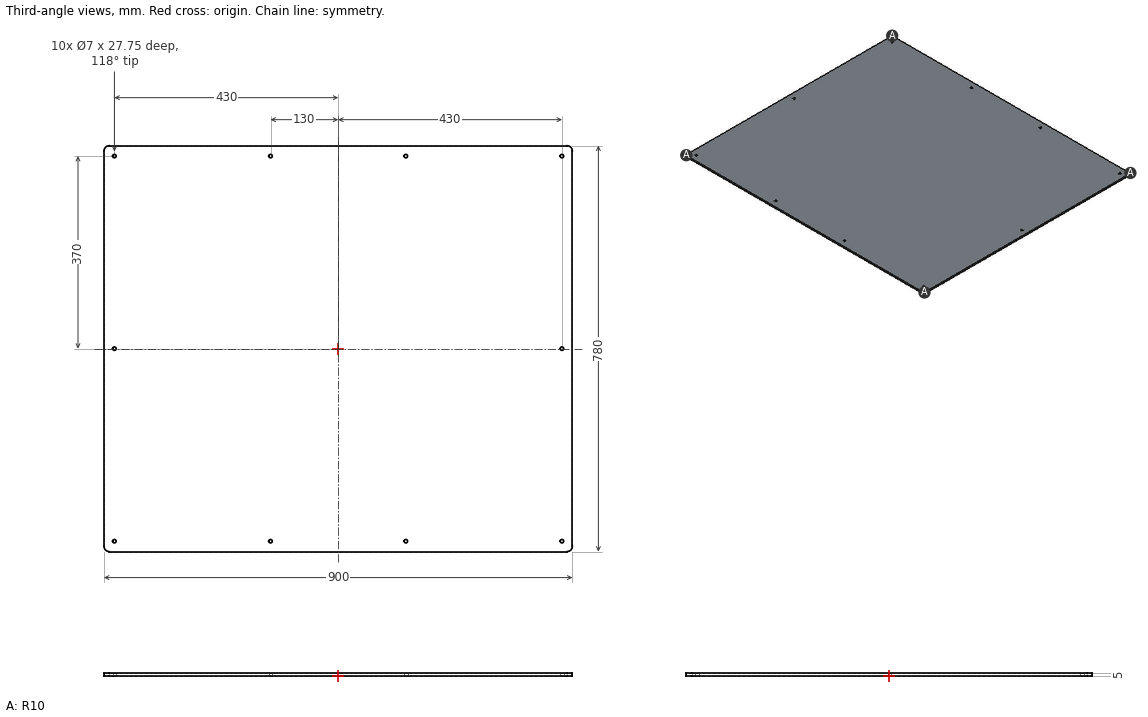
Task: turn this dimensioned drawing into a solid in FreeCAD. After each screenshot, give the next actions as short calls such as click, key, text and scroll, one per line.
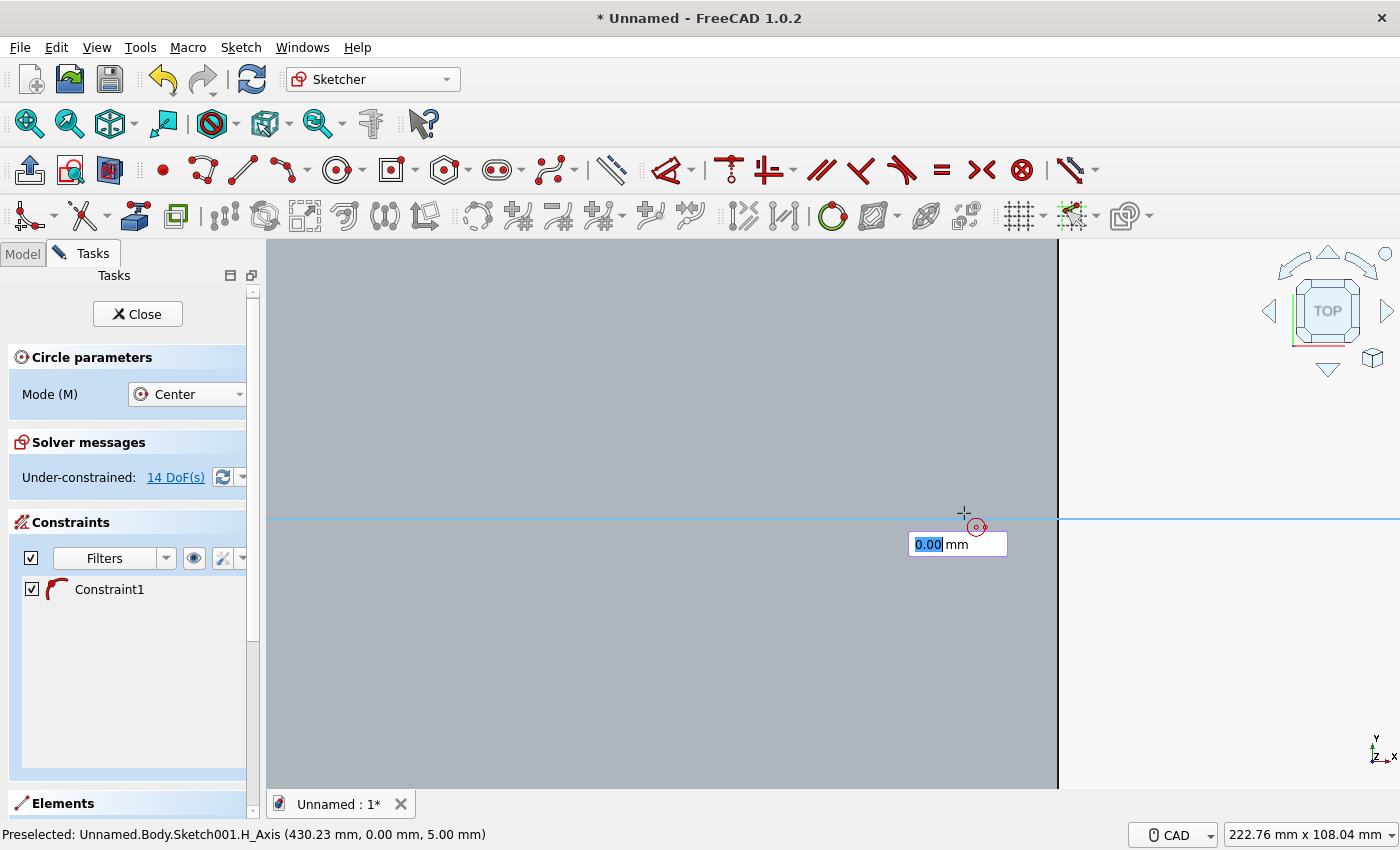
click(963, 503)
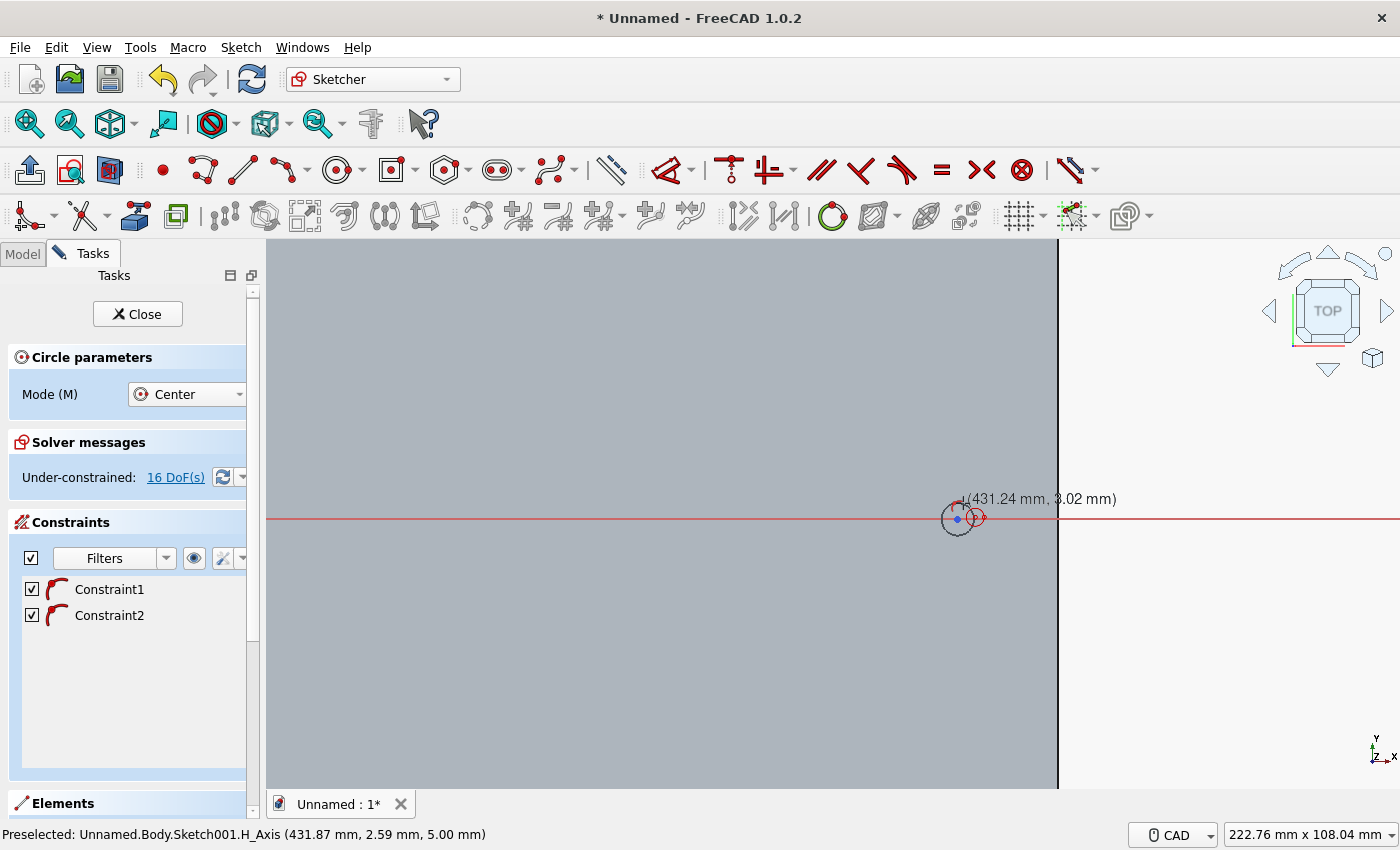
scroll(964, 513, down, 12)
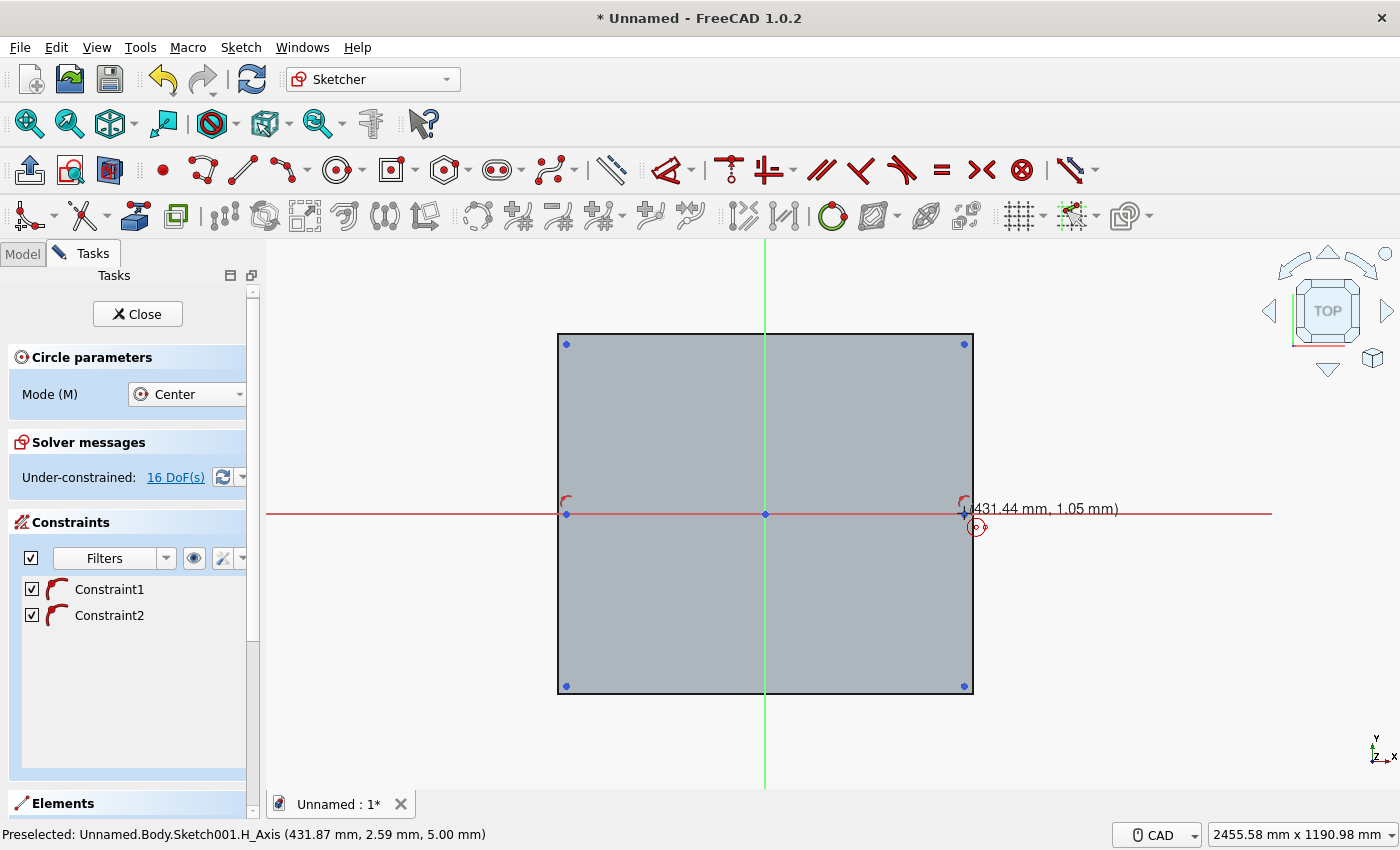
scroll(705, 343, up, 14)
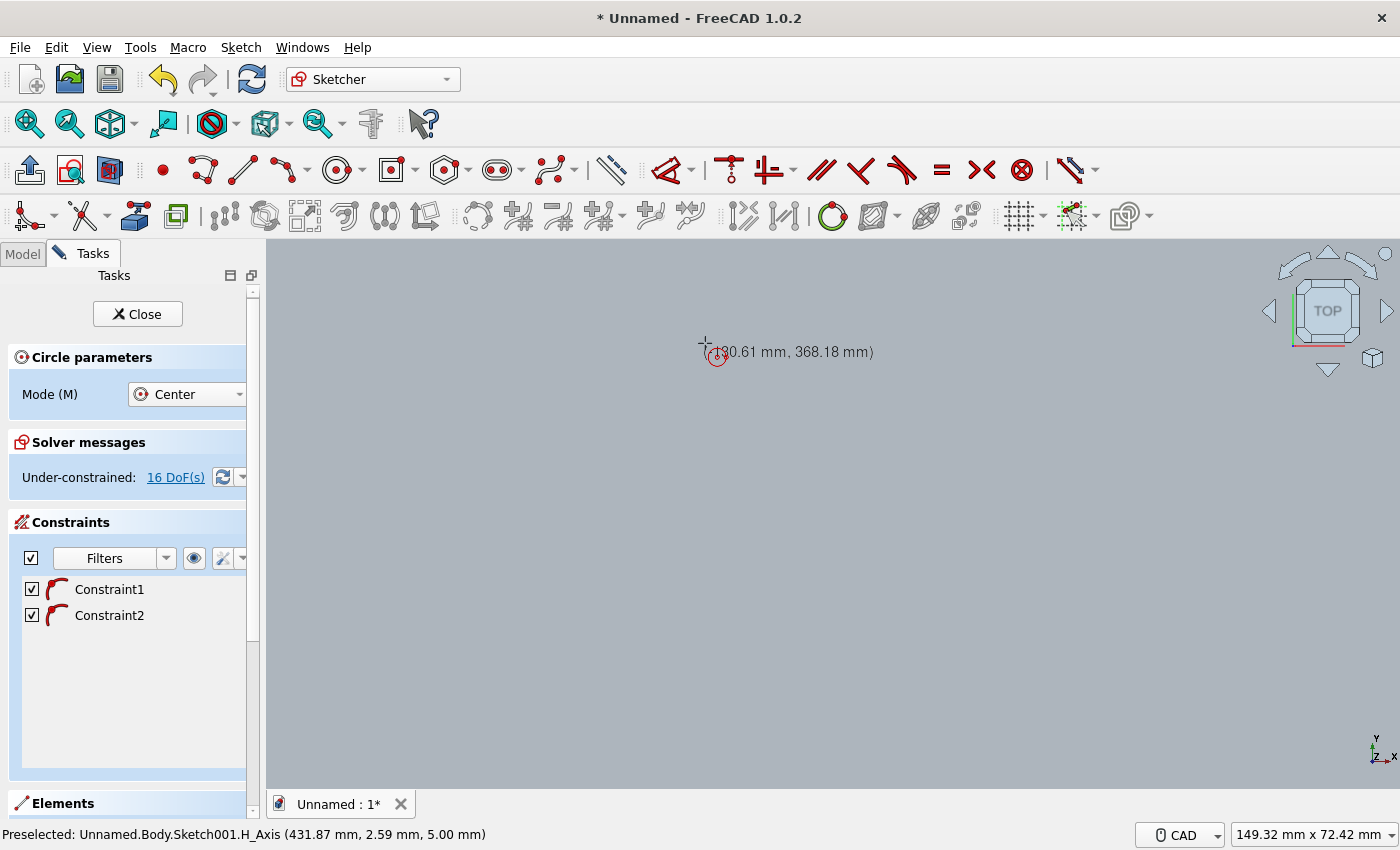
scroll(705, 343, down, 14)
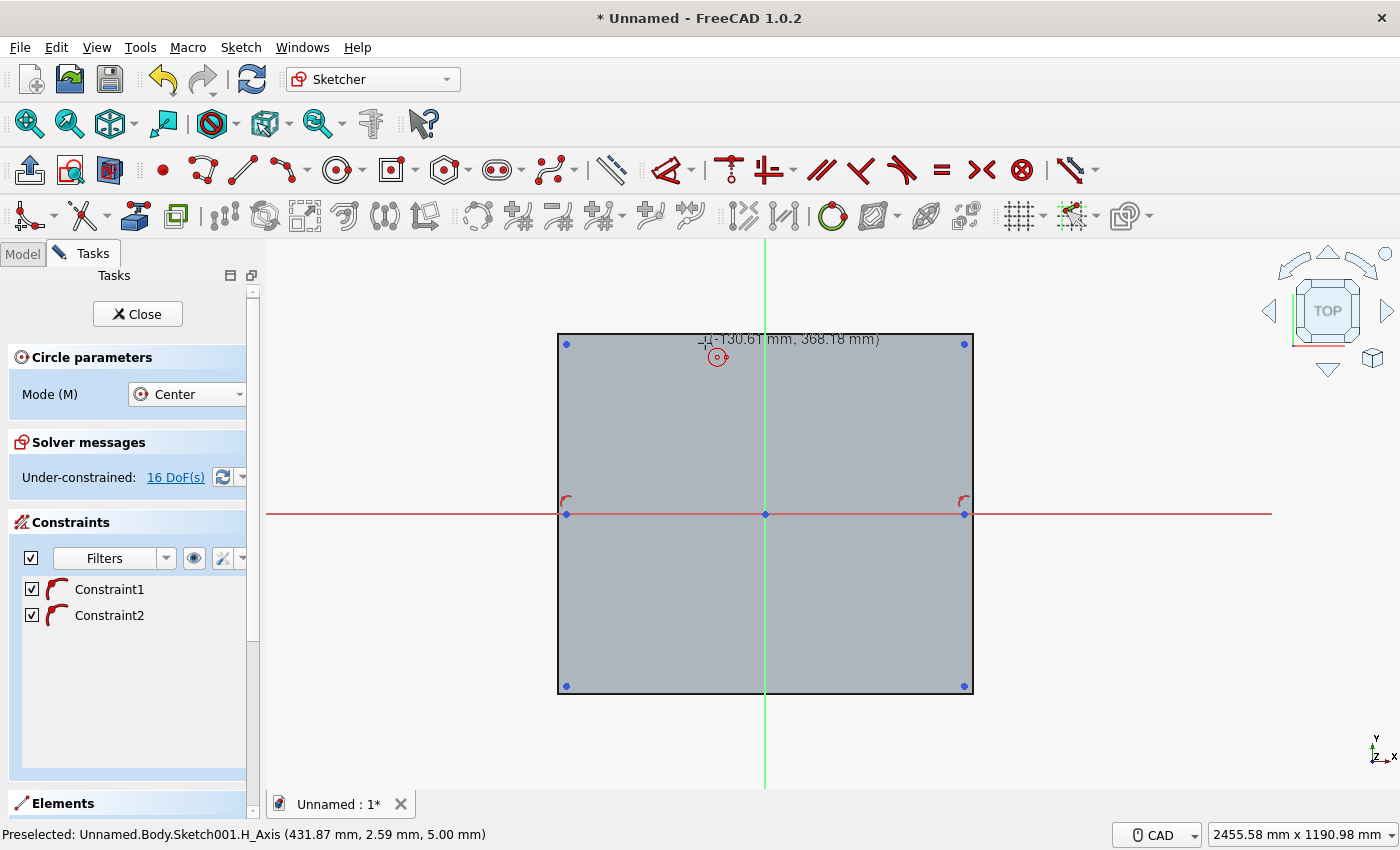
click(705, 343)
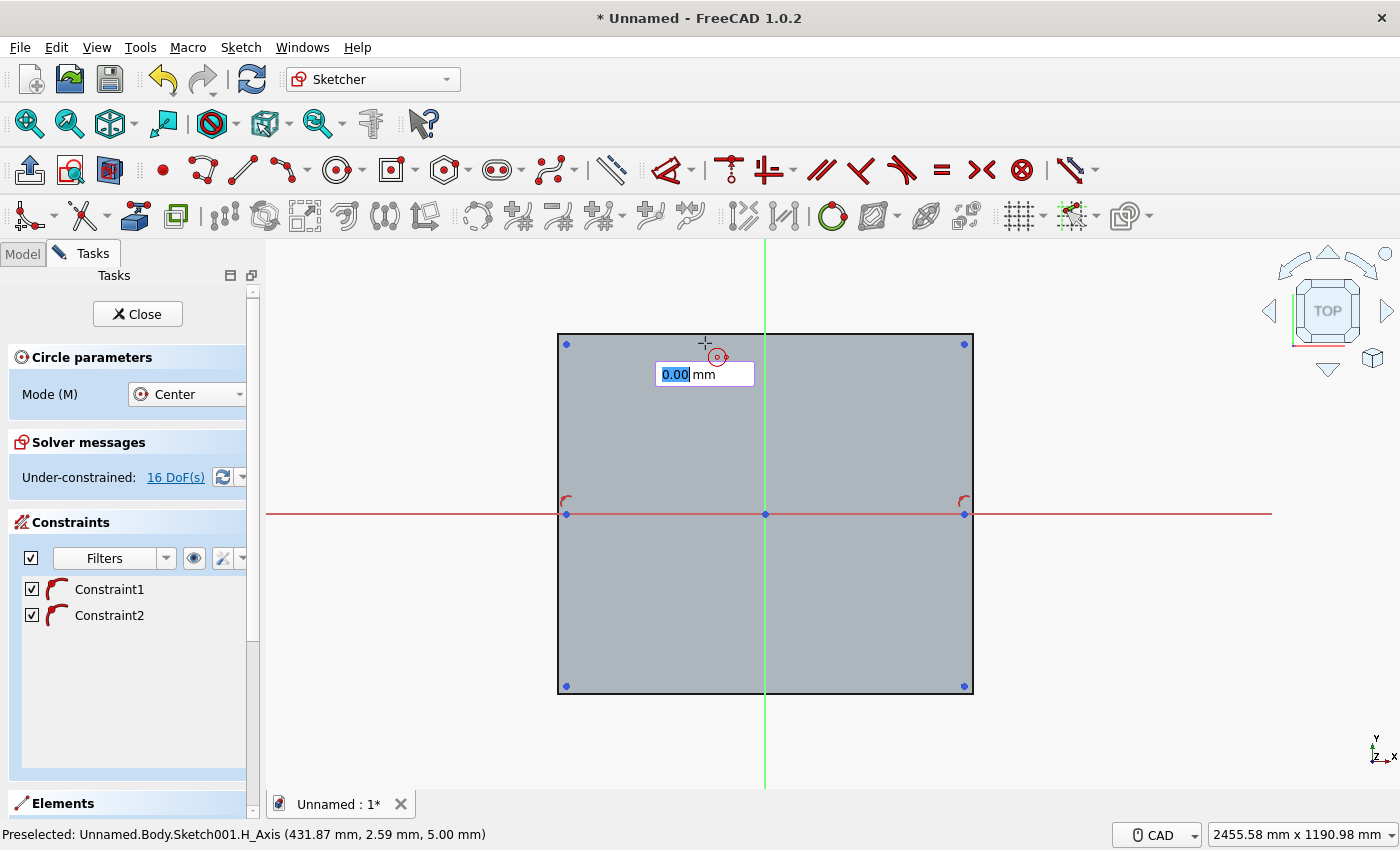
scroll(706, 342, up, 12)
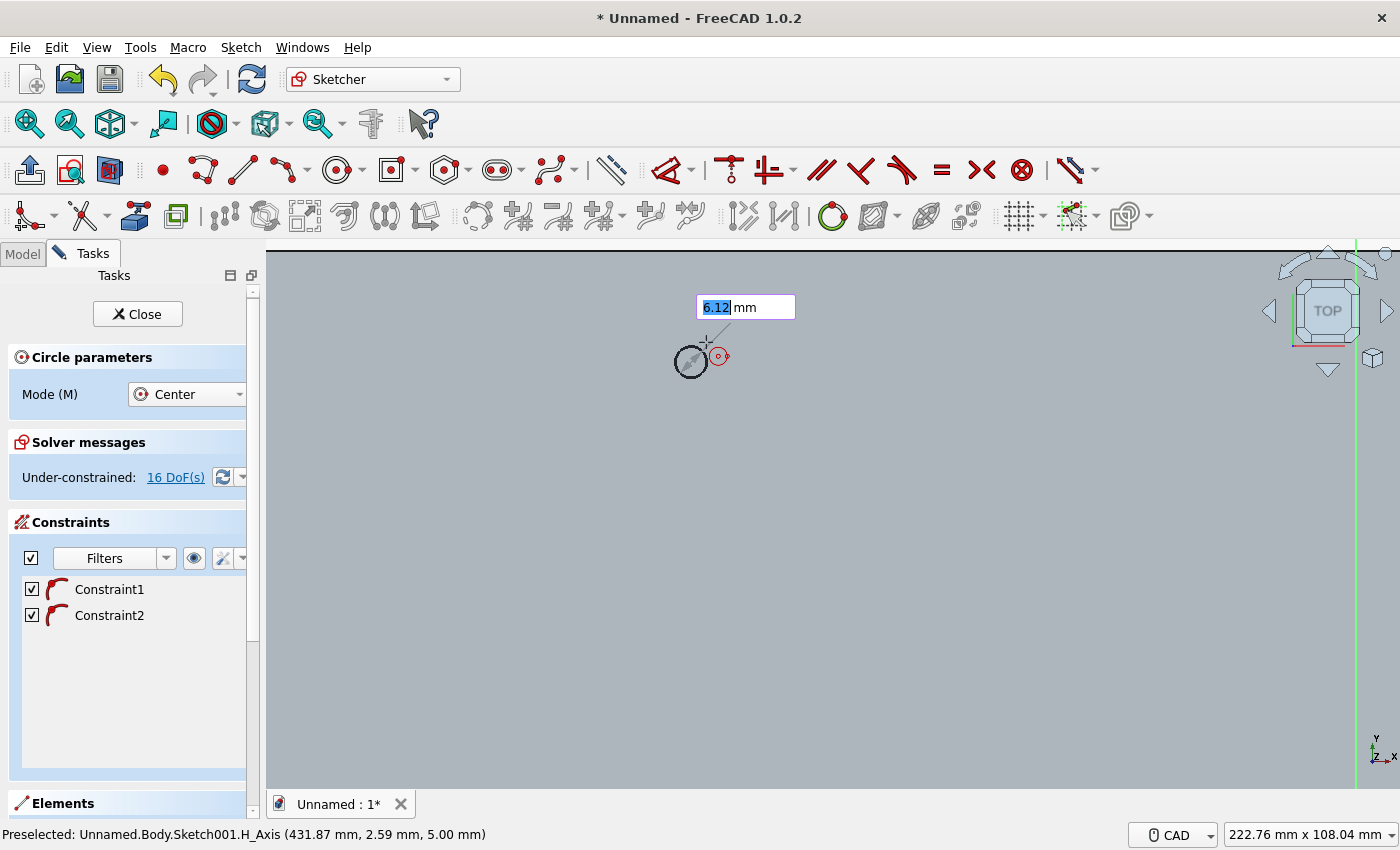
click(707, 340)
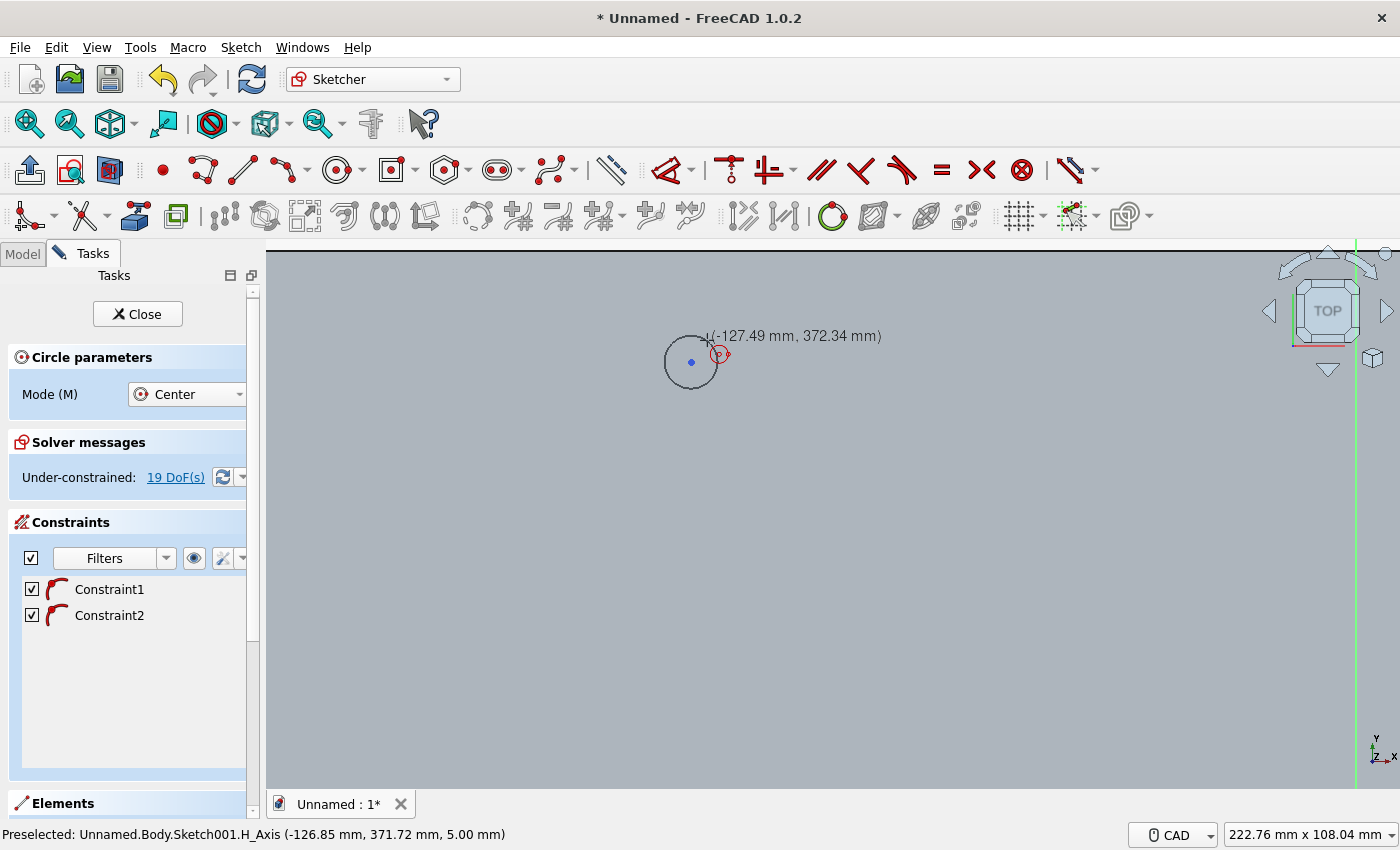
scroll(705, 342, down, 12)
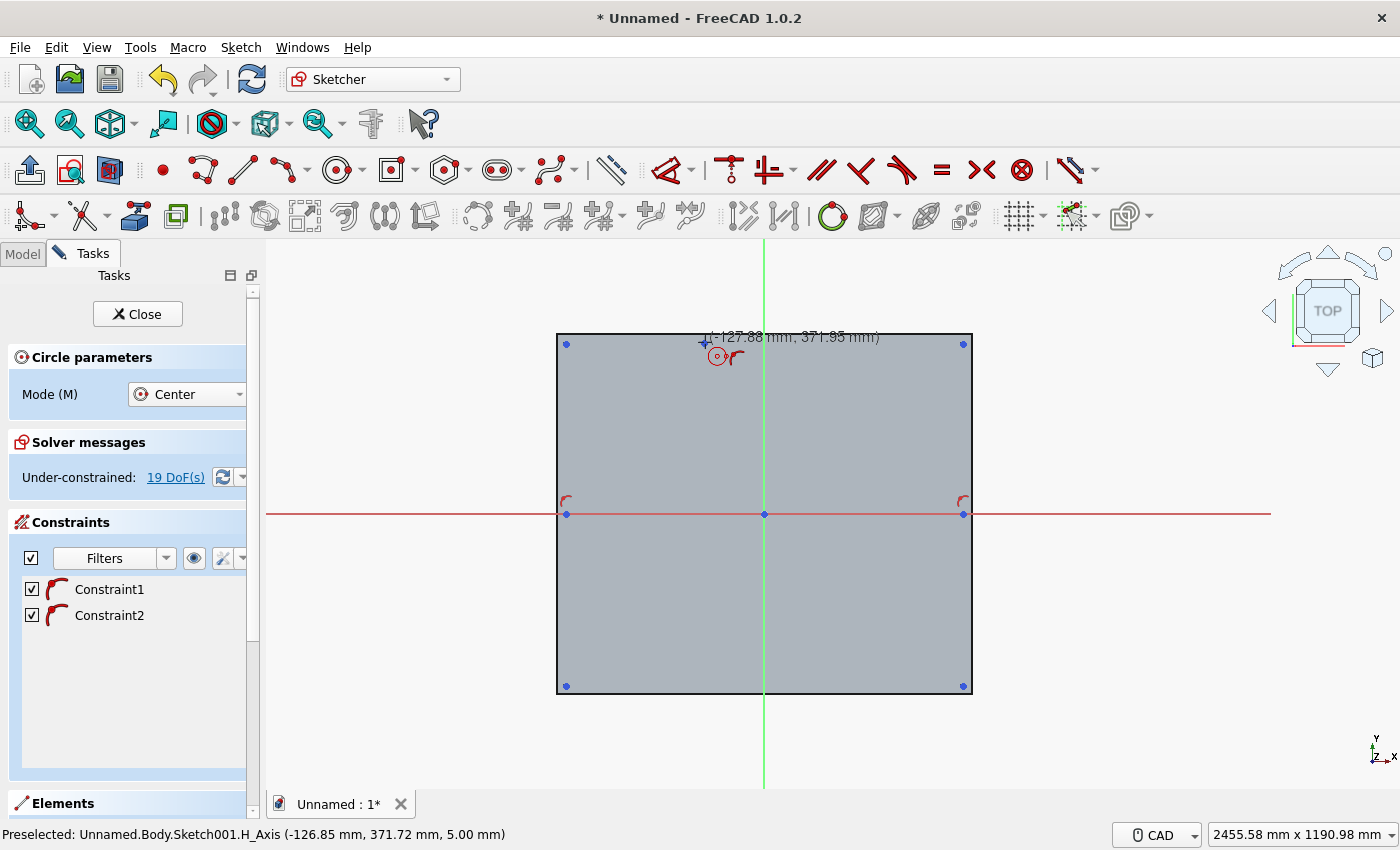
scroll(824, 343, up, 14)